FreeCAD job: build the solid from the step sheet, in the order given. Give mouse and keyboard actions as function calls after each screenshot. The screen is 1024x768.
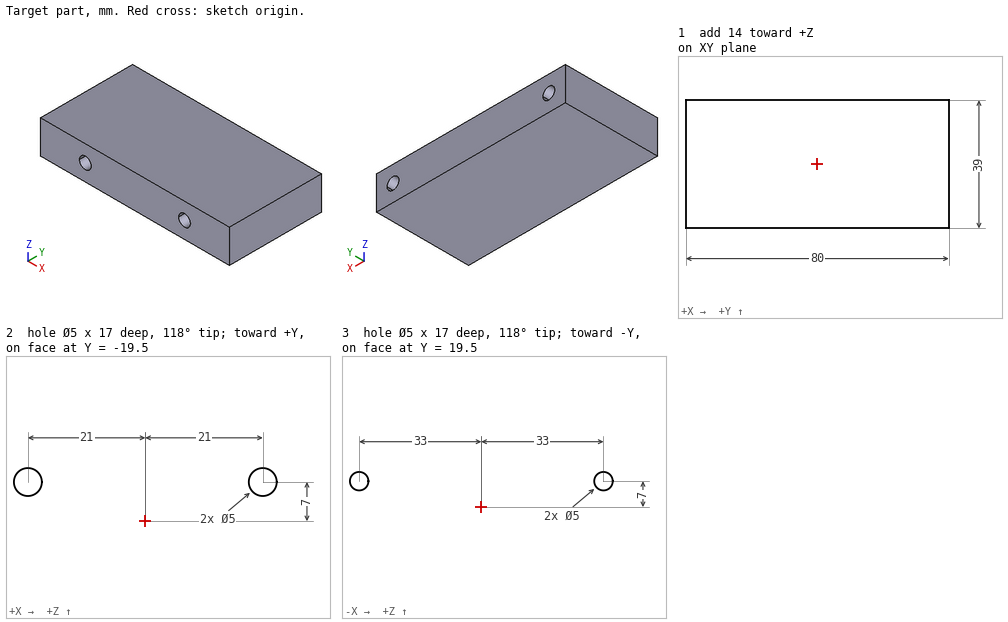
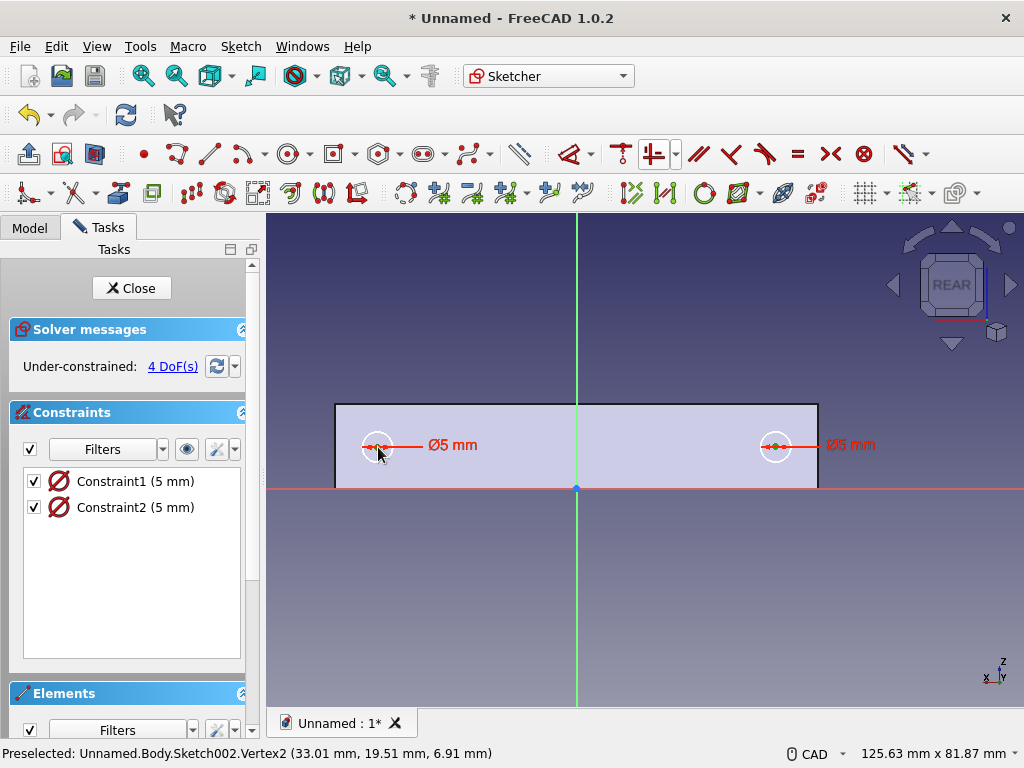
click(676, 154)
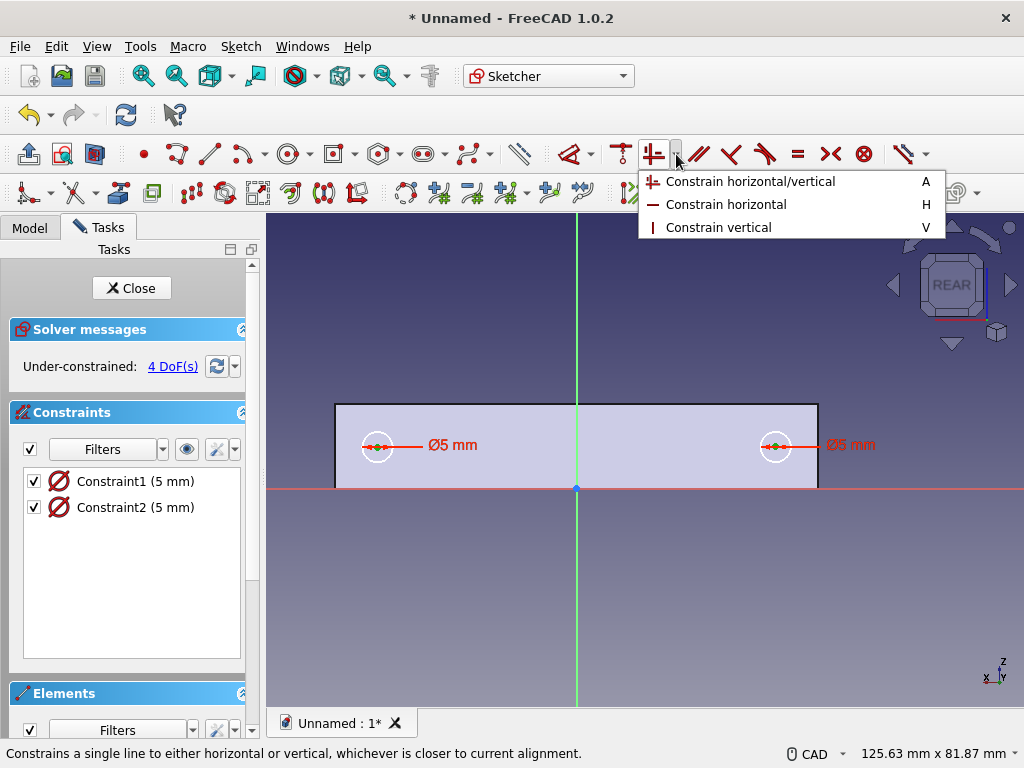
click(792, 204)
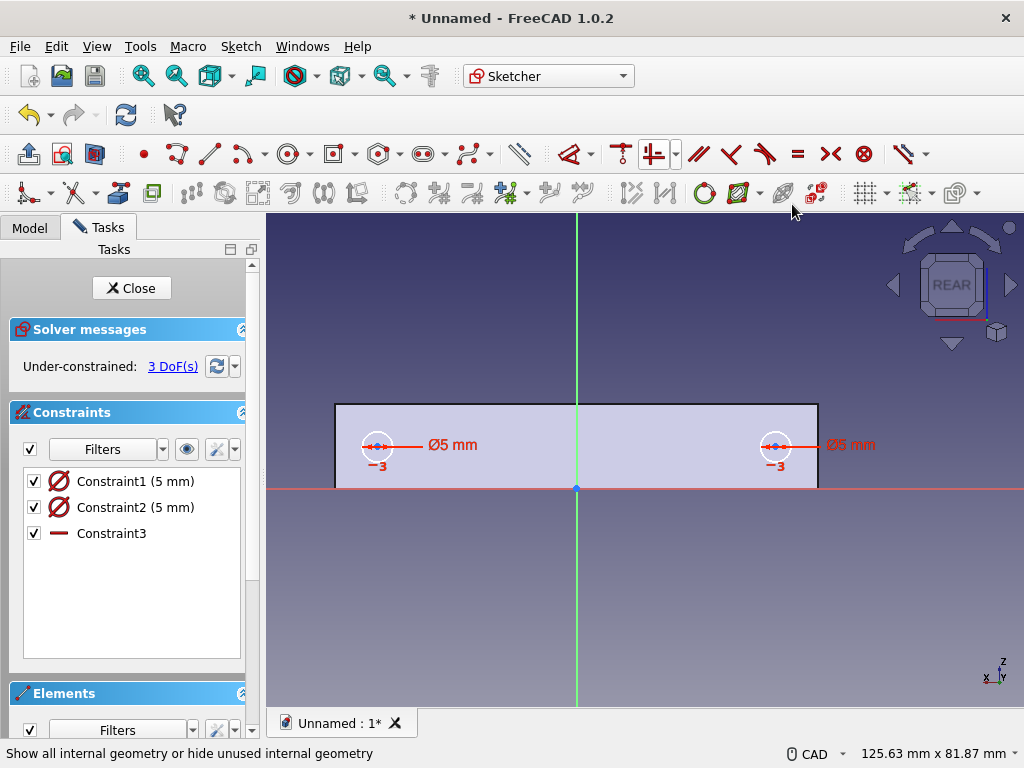
key(d)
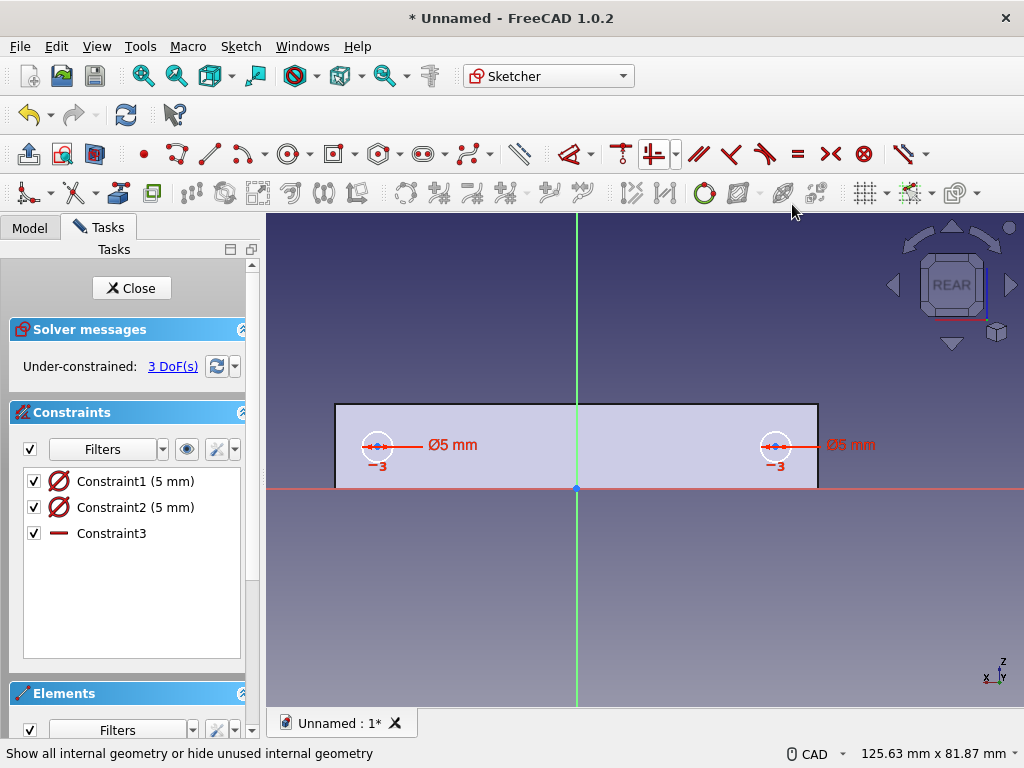
click(776, 447)
click(810, 468)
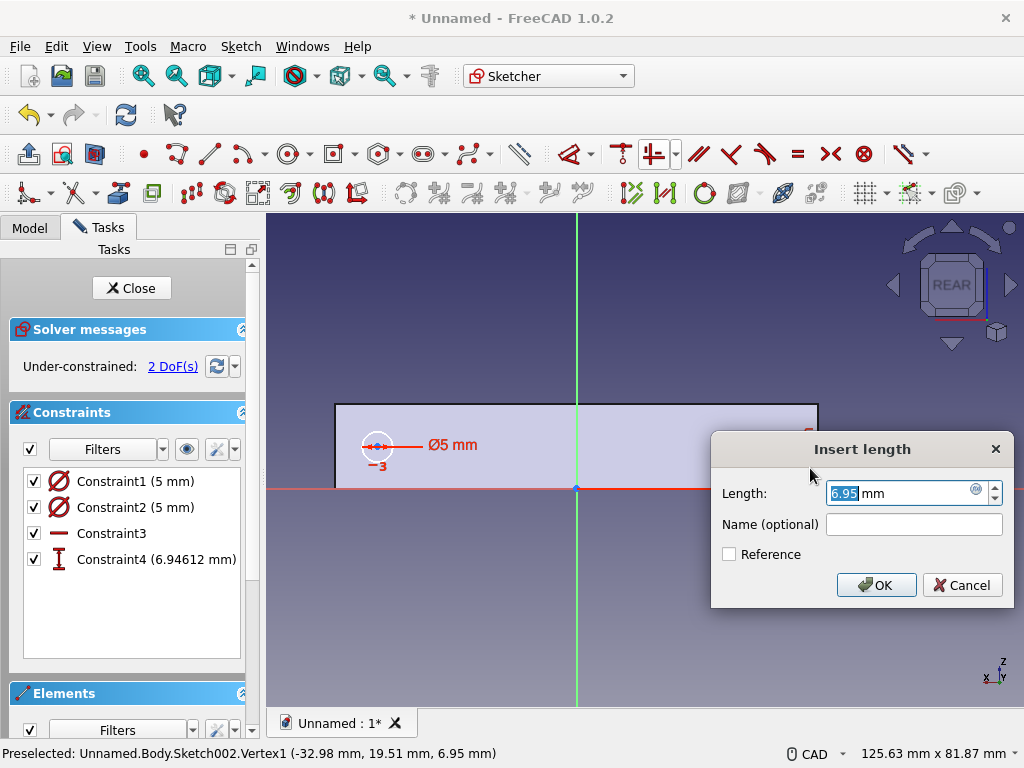
text(7)
key(Return)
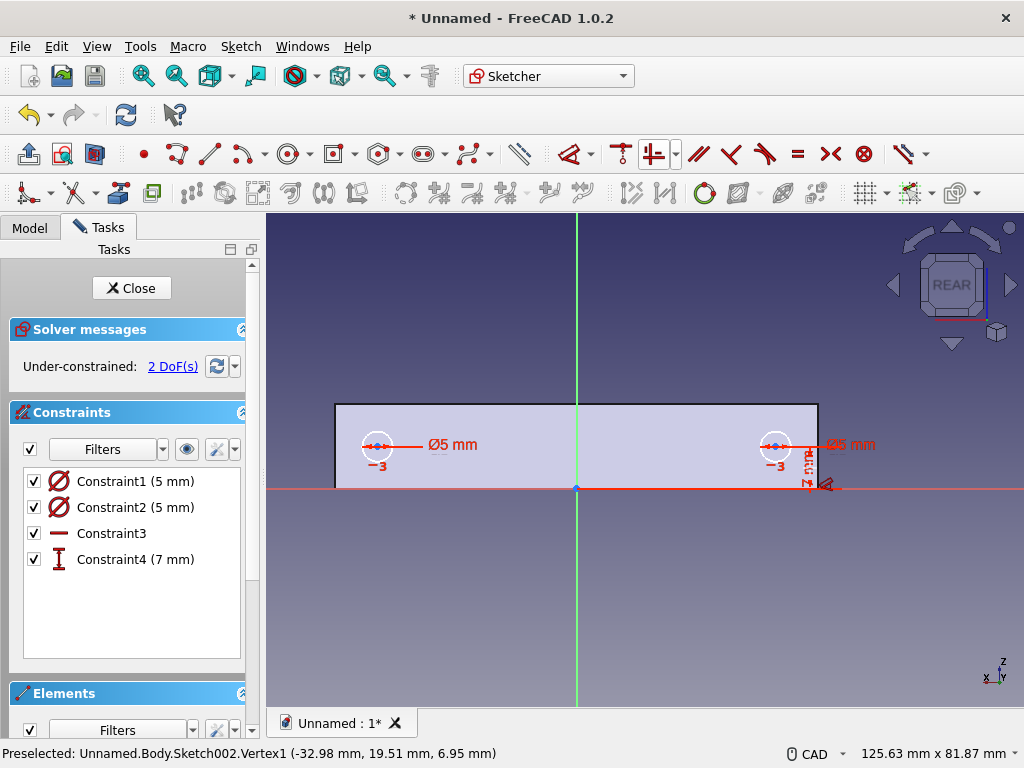
click(776, 447)
click(676, 523)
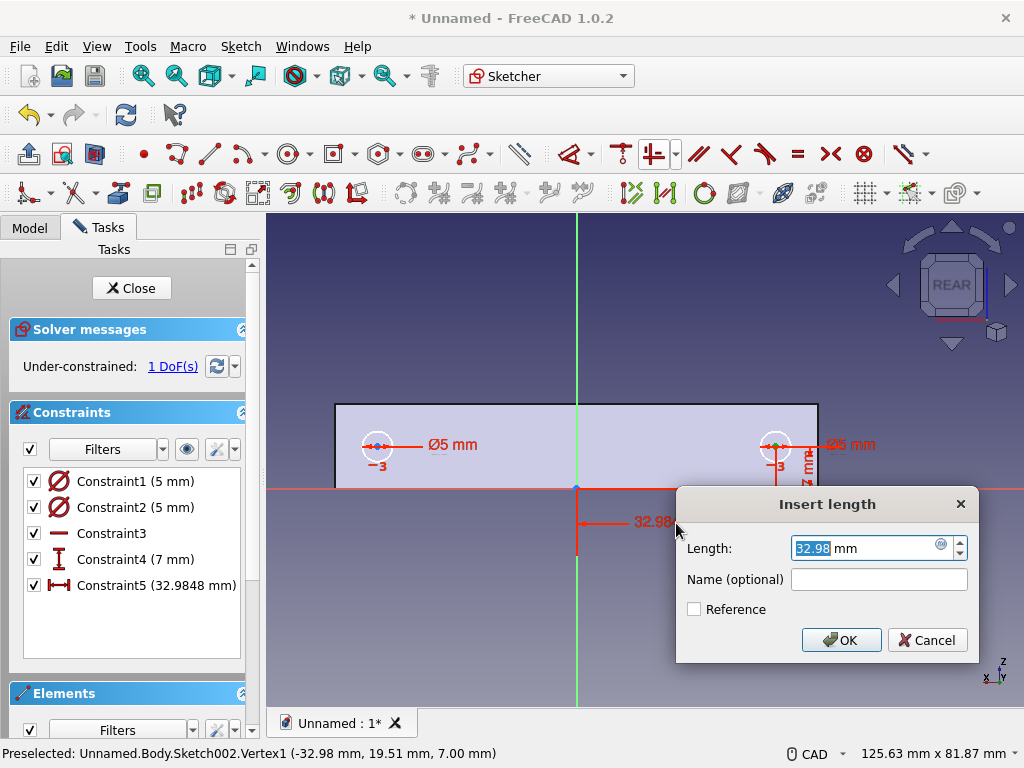
text(33)
key(Return)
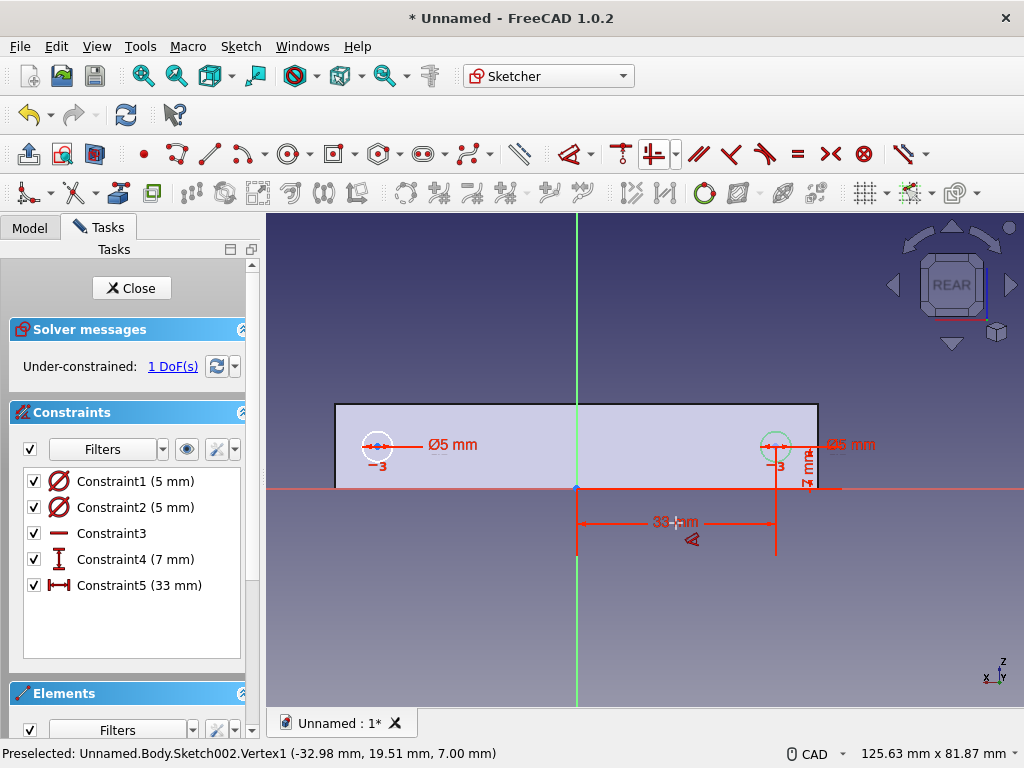
click(378, 447)
click(477, 523)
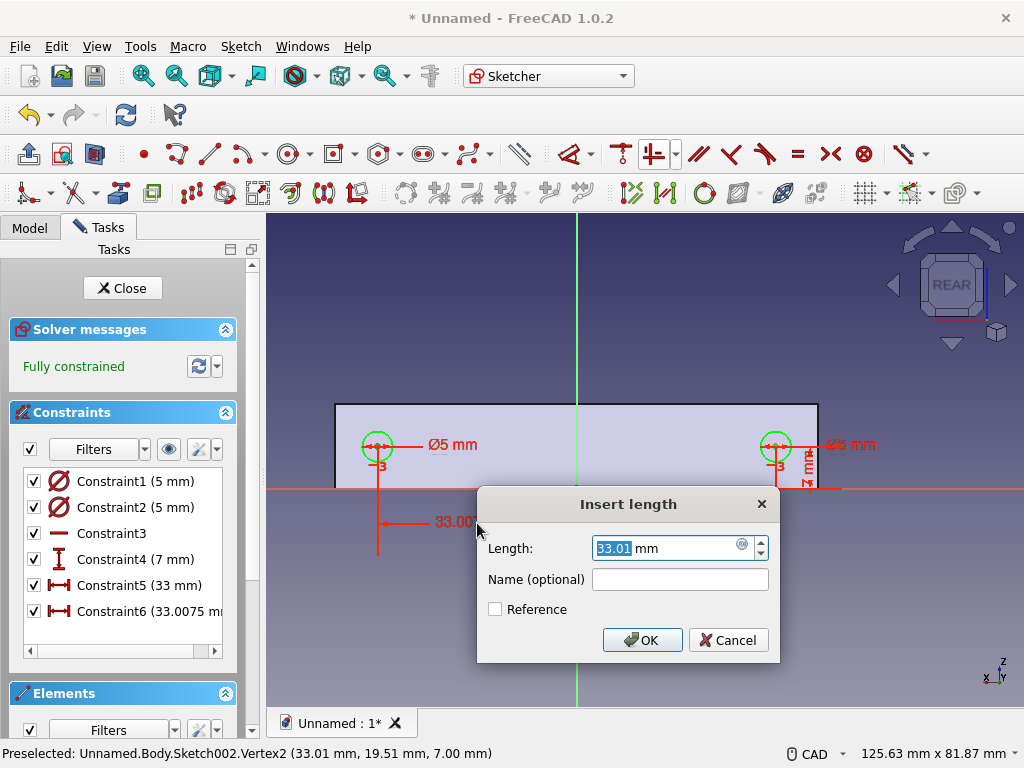
text(33)
key(Return)
key(Escape)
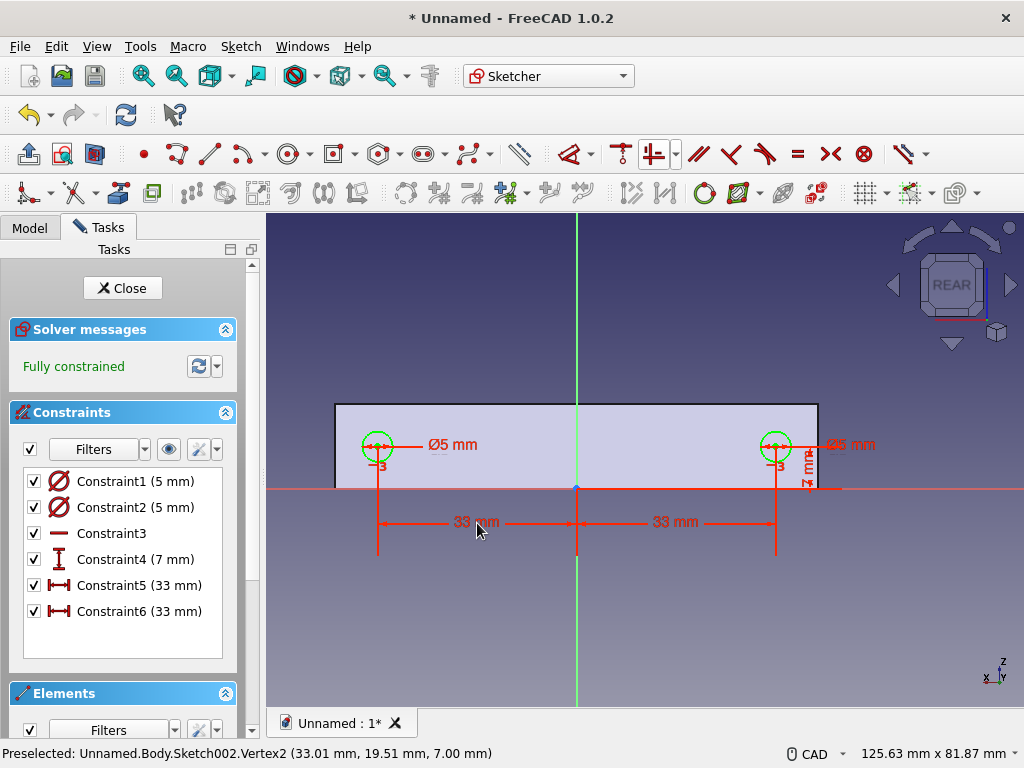
click(123, 288)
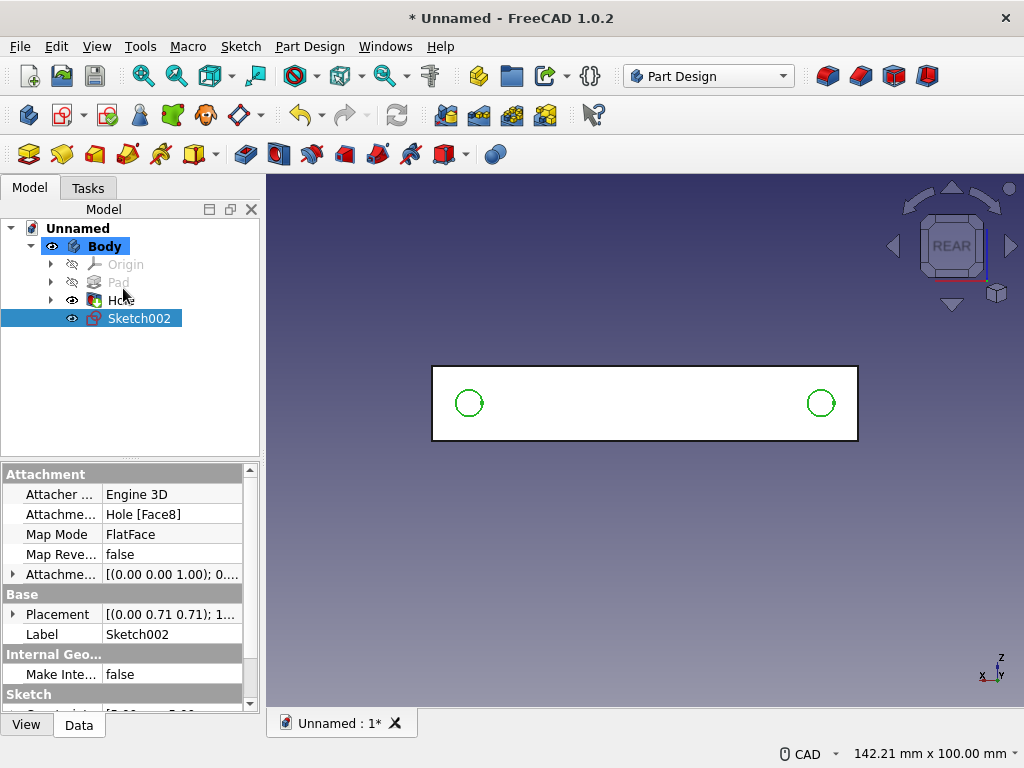
click(279, 154)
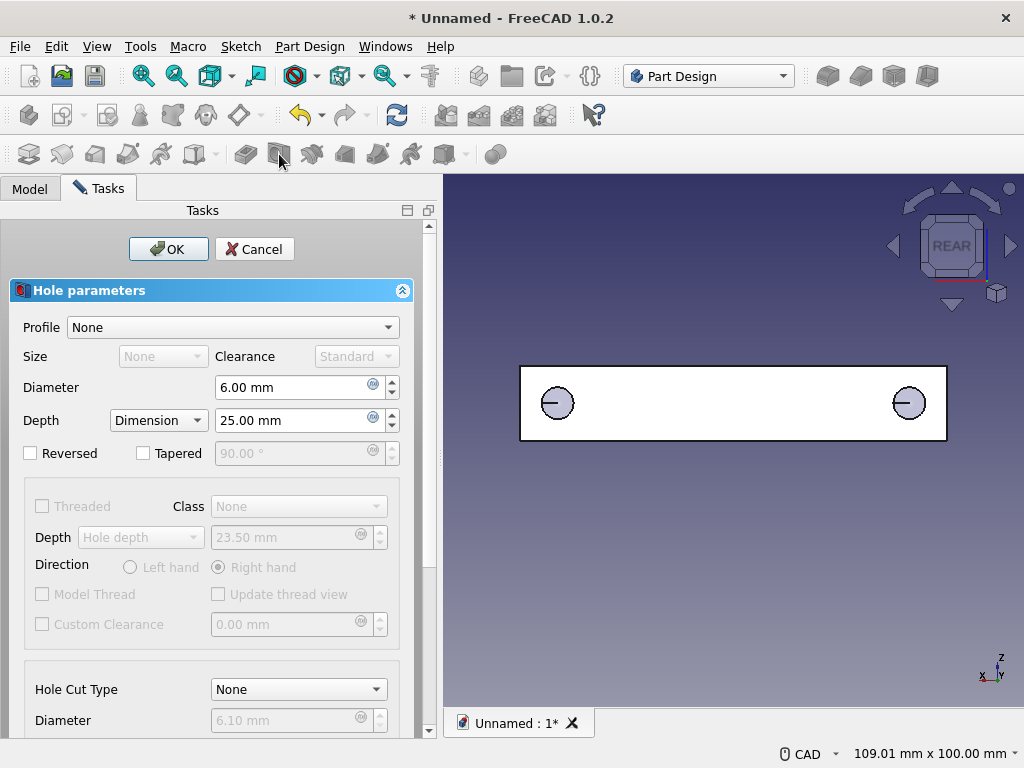
triple_click(300, 388)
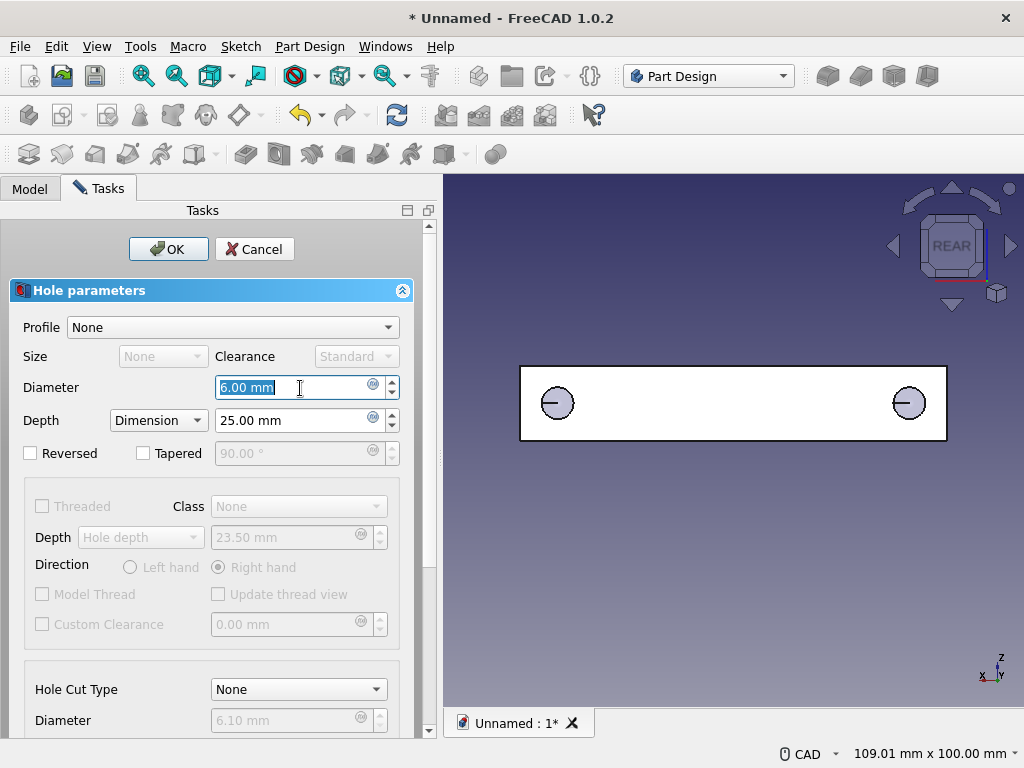
text(5)
key(Tab)